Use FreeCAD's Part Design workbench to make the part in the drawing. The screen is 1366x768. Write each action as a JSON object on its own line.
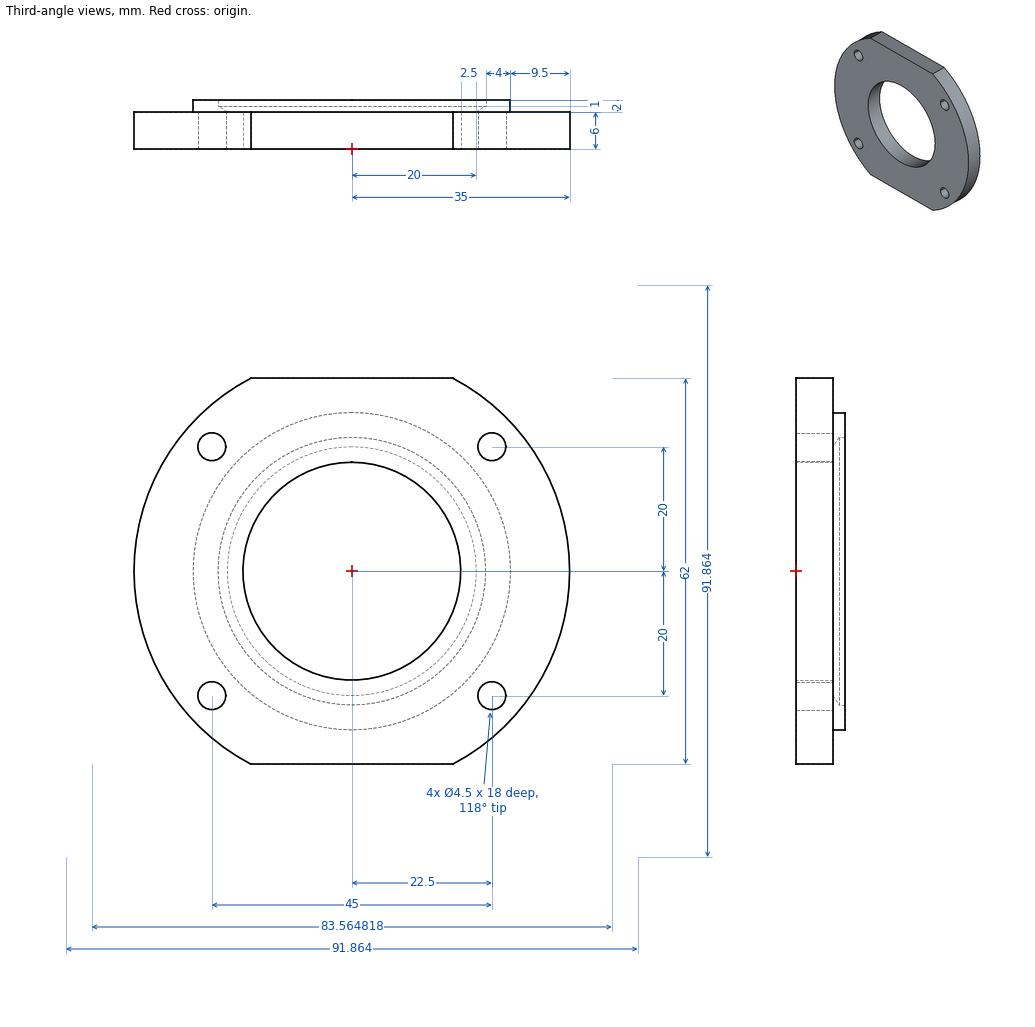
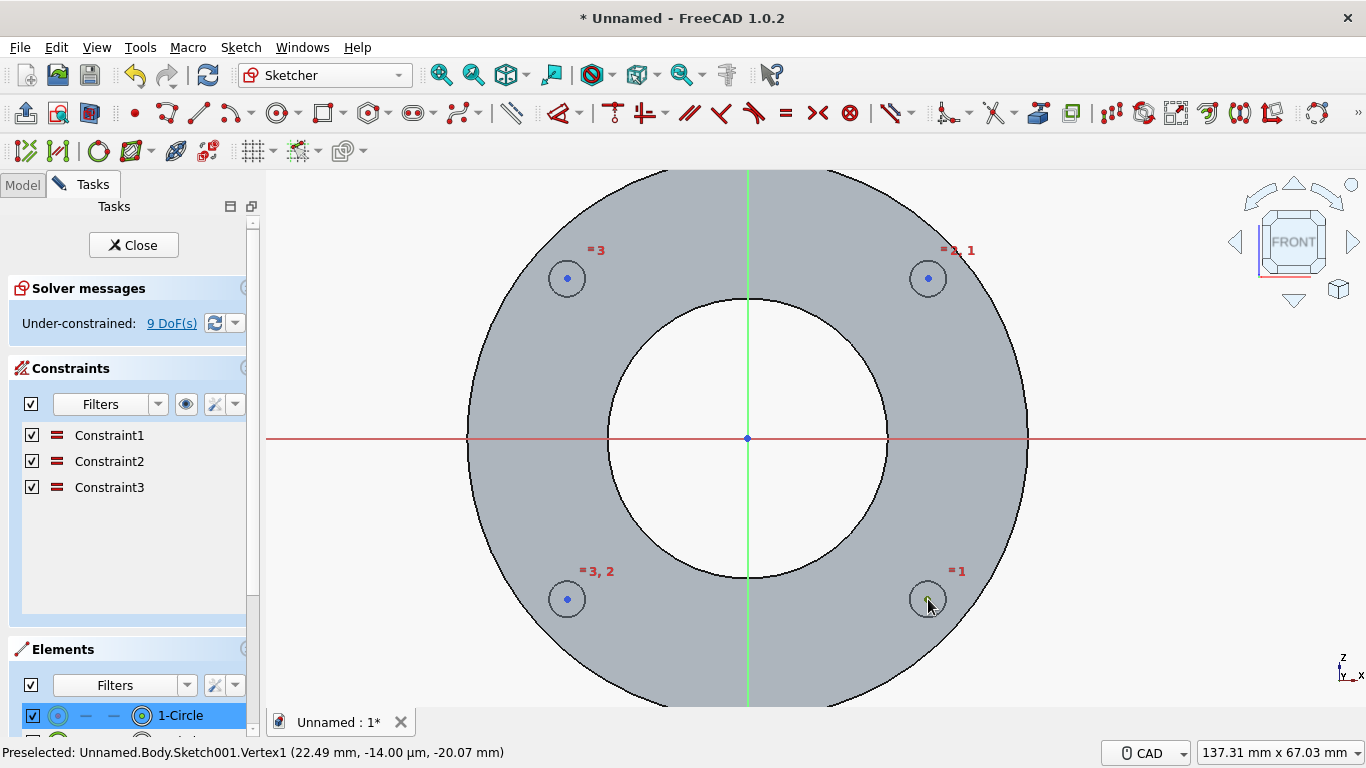
{"action": "left_click", "coordinate": [928, 279]}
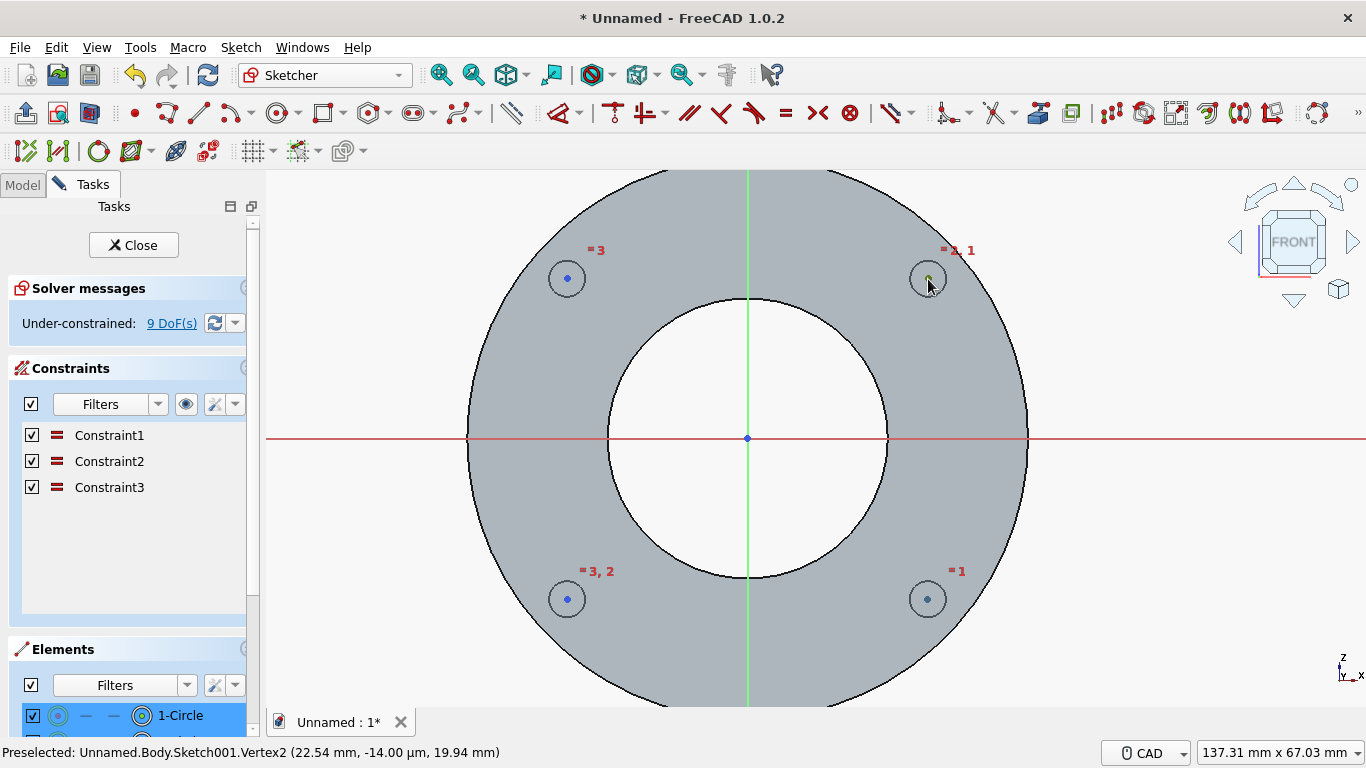
{"action": "left_click", "coordinate": [668, 114]}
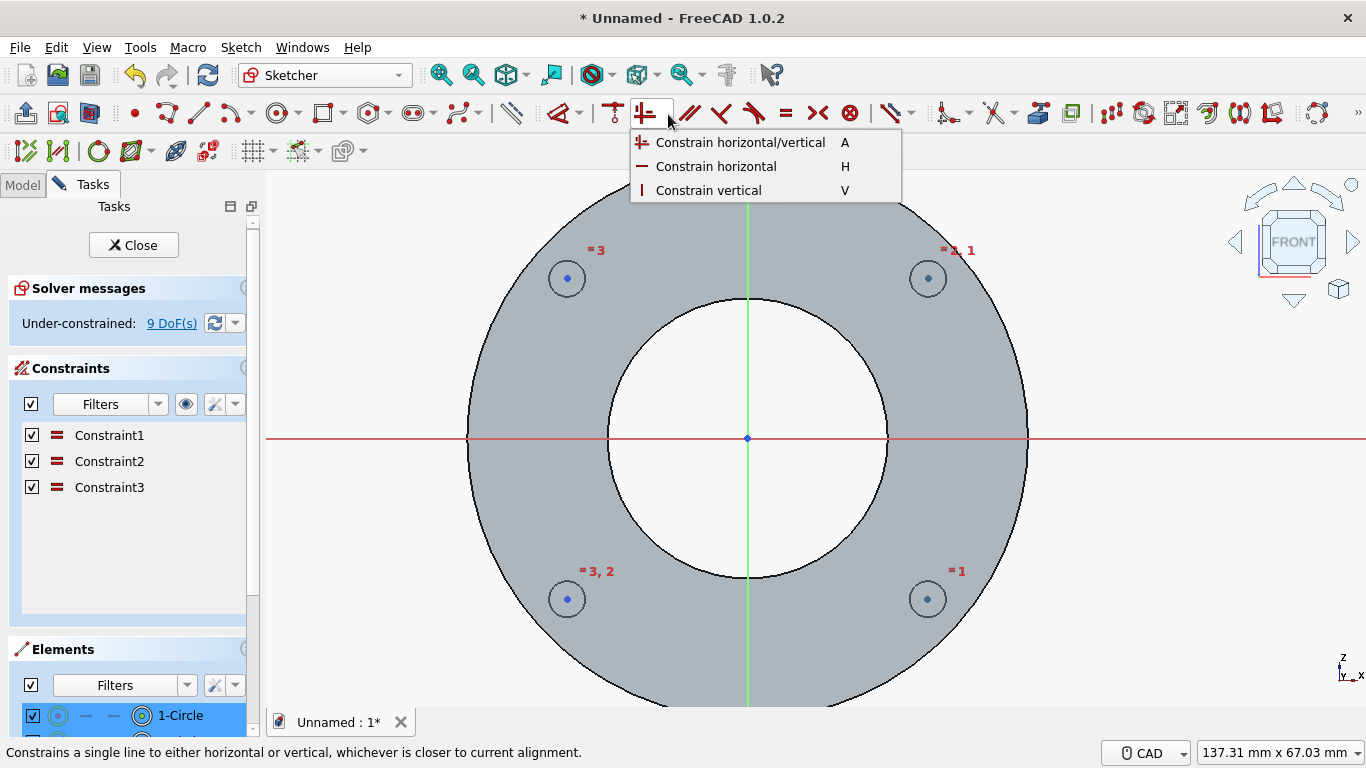
{"action": "left_click", "coordinate": [766, 190]}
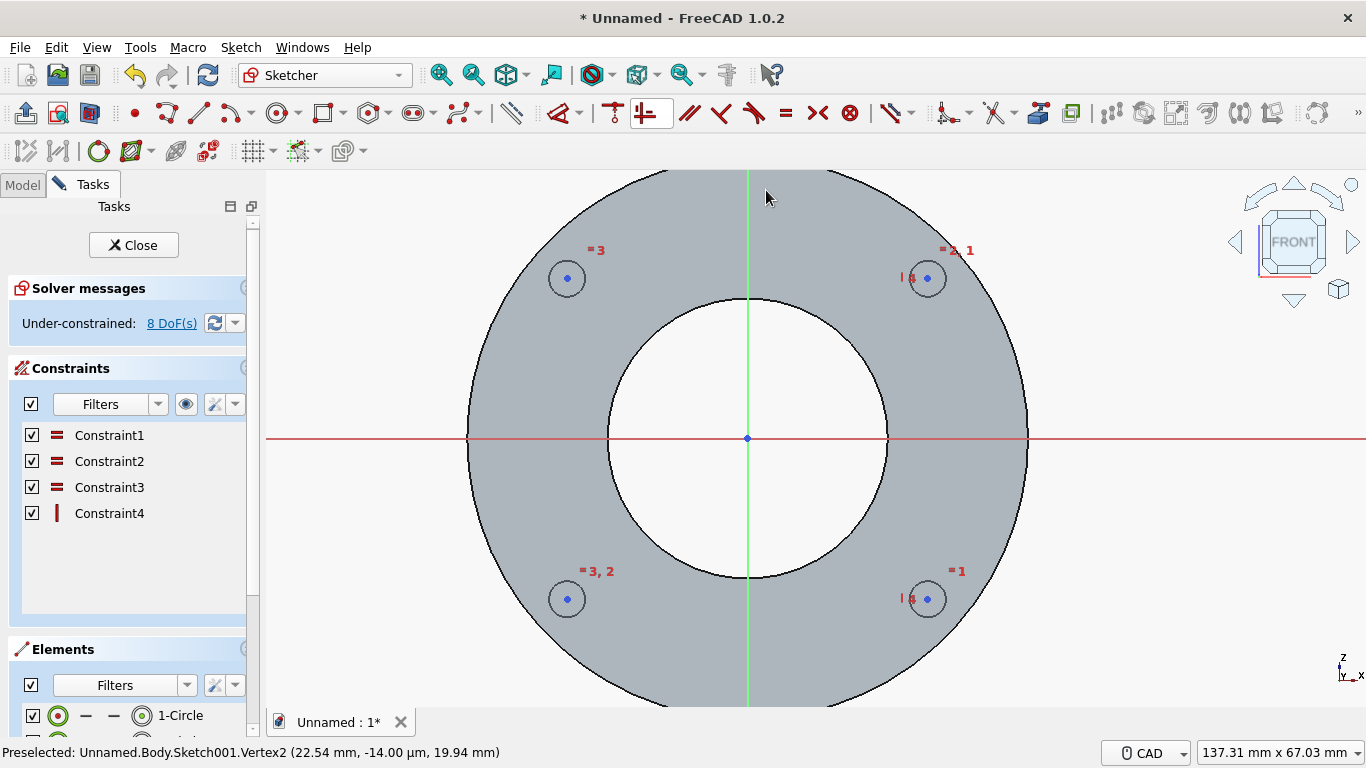
{"action": "left_click", "coordinate": [928, 599]}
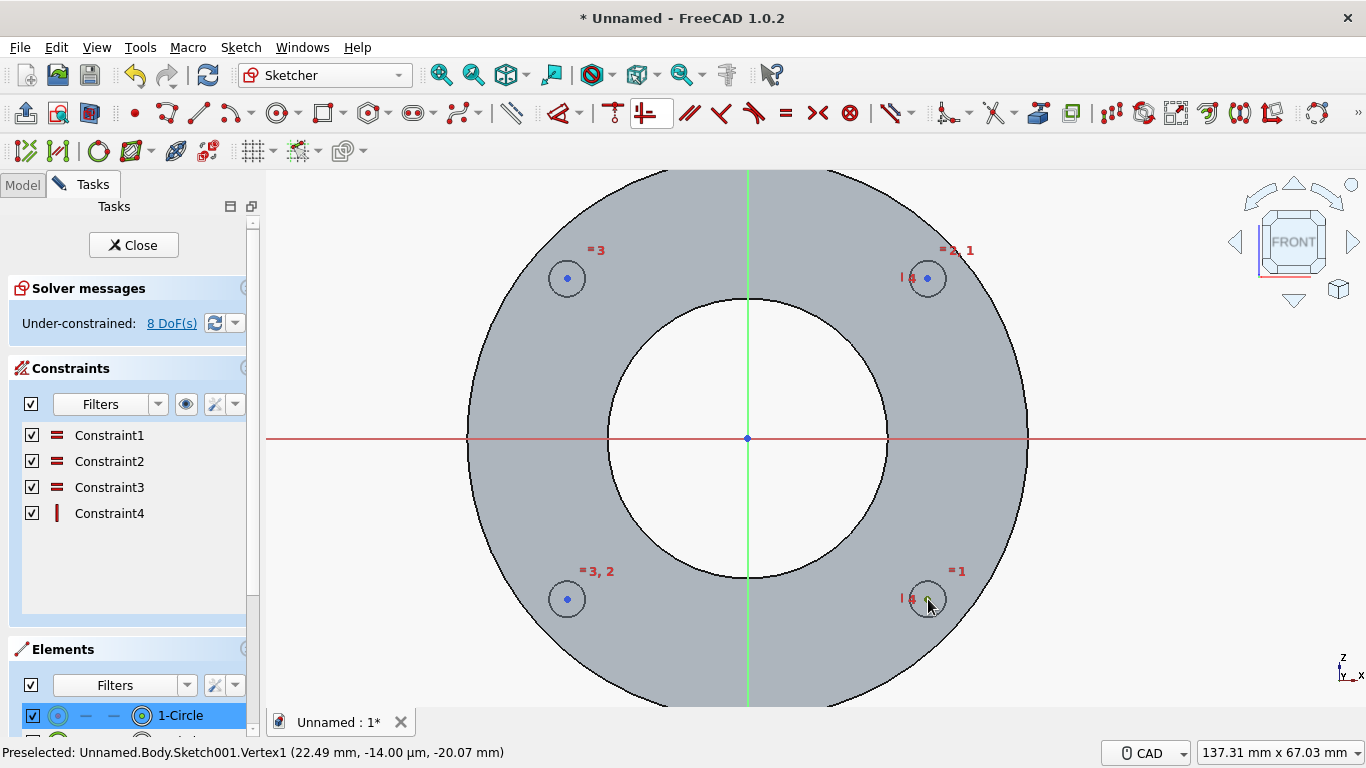
{"action": "left_click", "coordinate": [567, 599]}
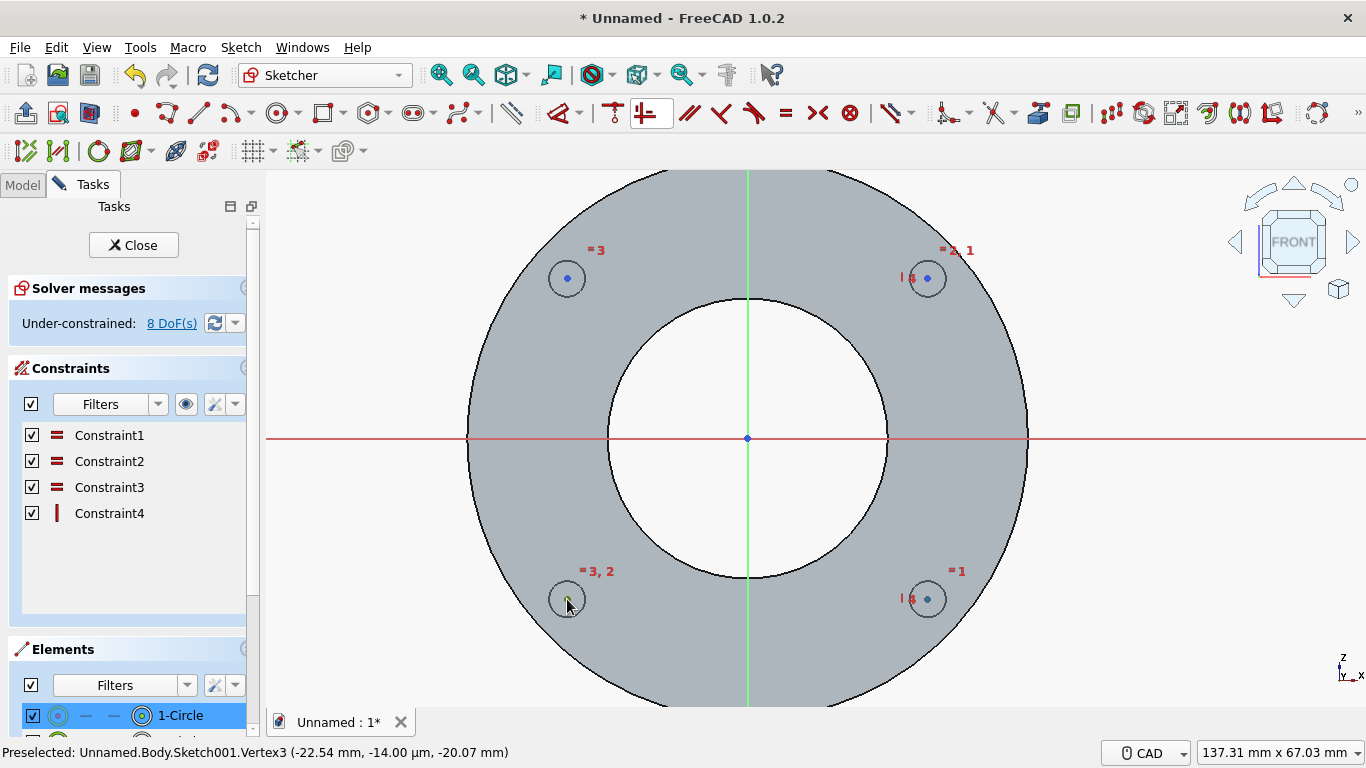
{"action": "left_click", "coordinate": [668, 114]}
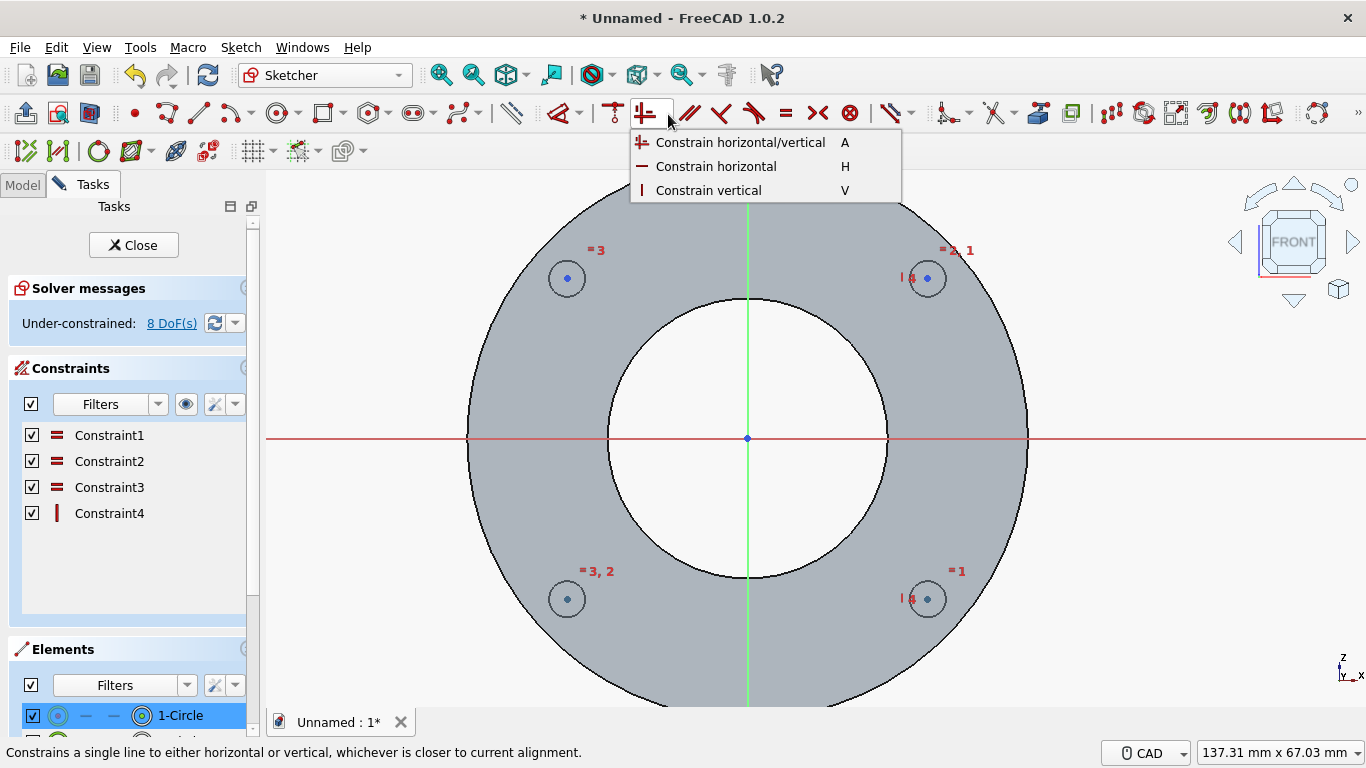
{"action": "left_click", "coordinate": [766, 166]}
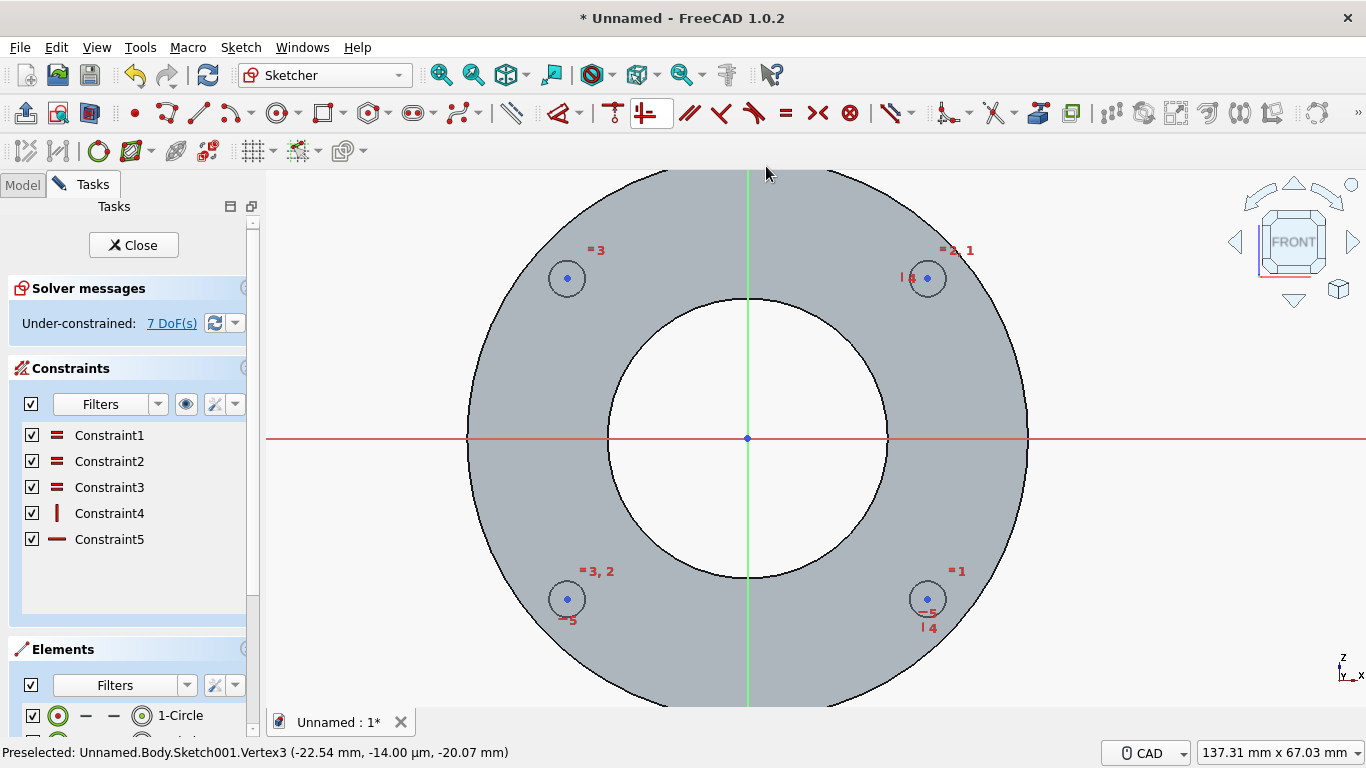
{"action": "left_click", "coordinate": [567, 599]}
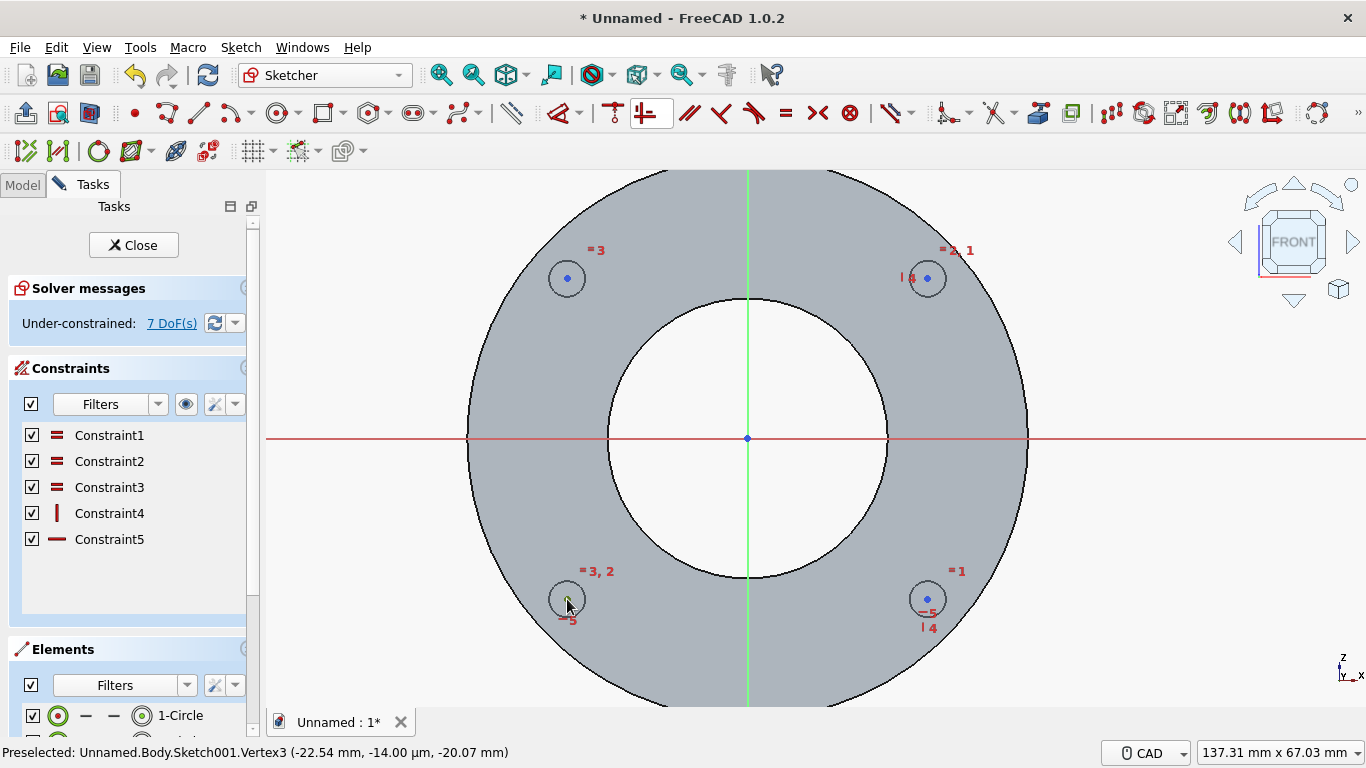
{"action": "left_click", "coordinate": [567, 279]}